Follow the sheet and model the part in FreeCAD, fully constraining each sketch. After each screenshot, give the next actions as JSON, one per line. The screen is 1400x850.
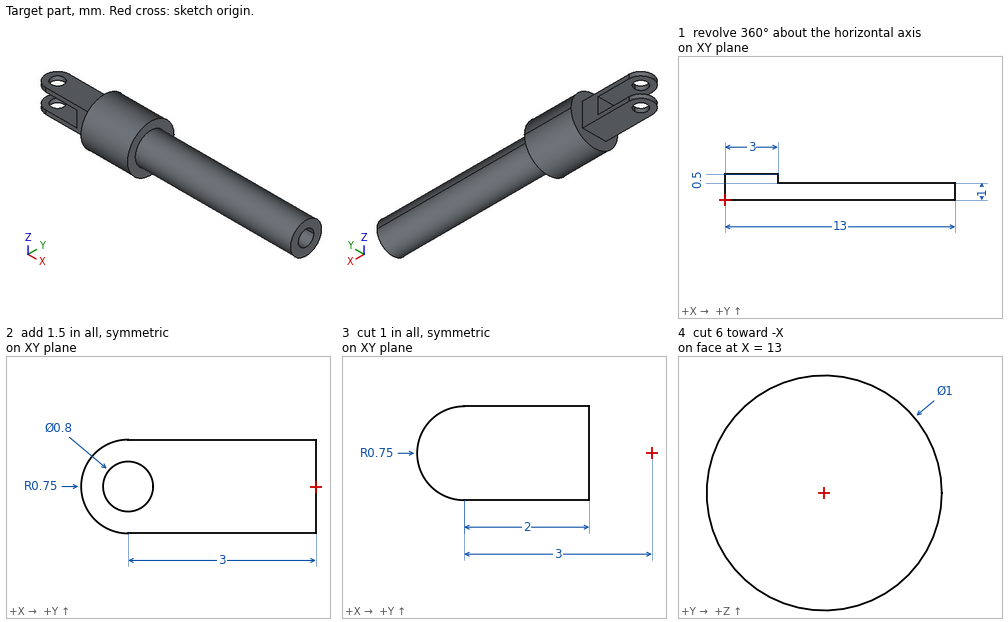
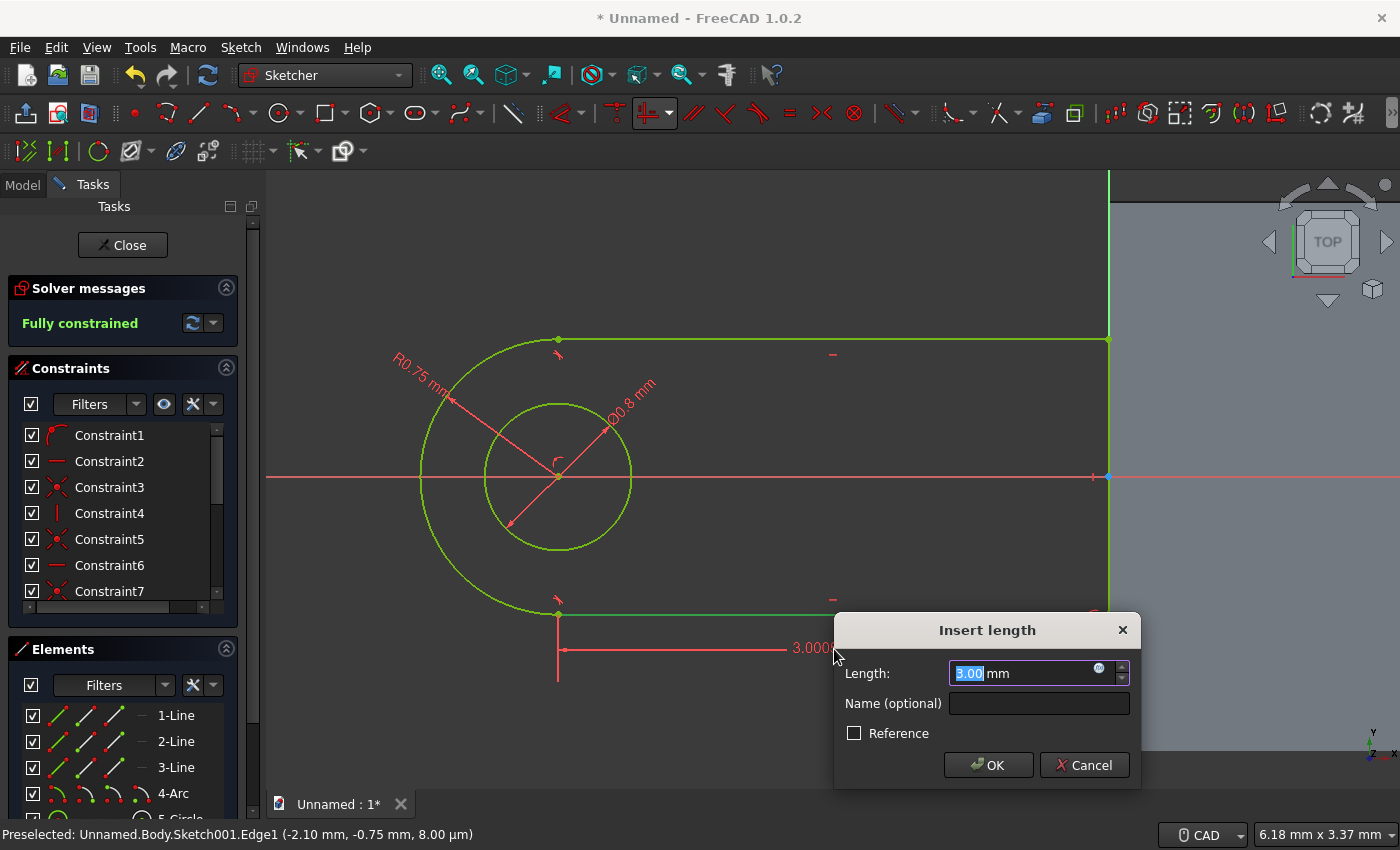
{"action": "type", "text": "3"}
{"action": "key", "text": "Return"}
{"action": "key", "text": "Escape"}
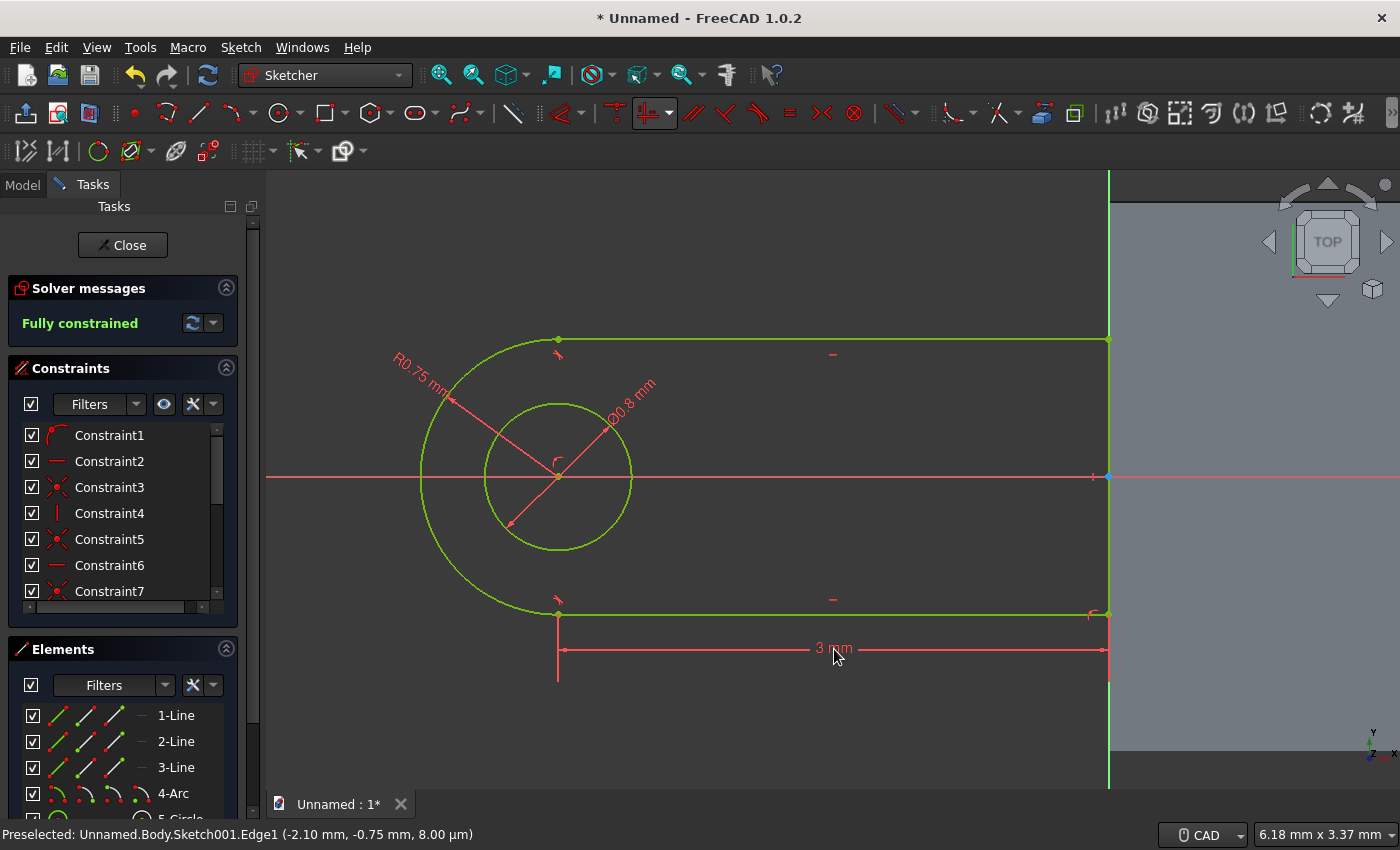
{"action": "left_click", "coordinate": [123, 245]}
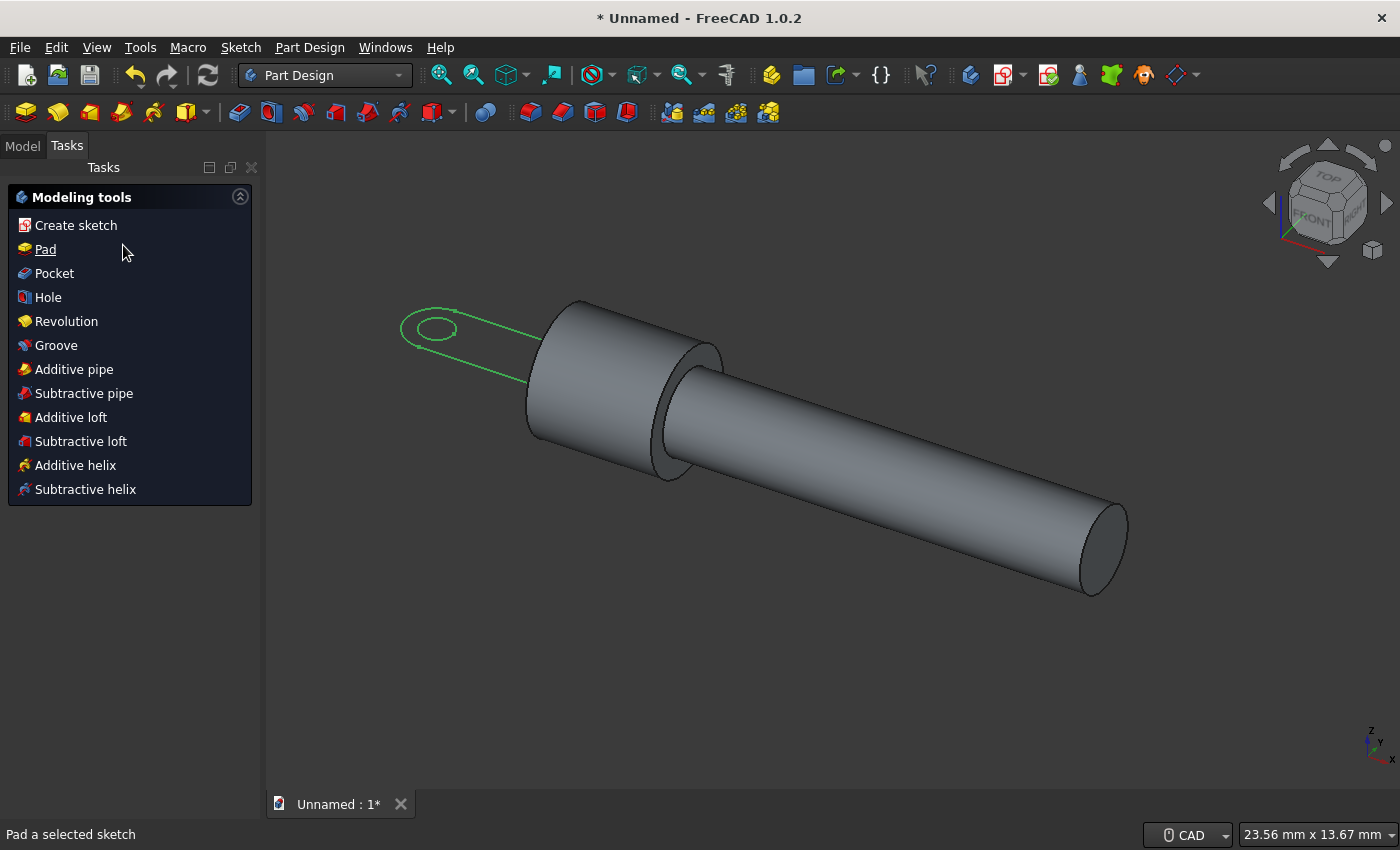
{"action": "left_click", "coordinate": [26, 112]}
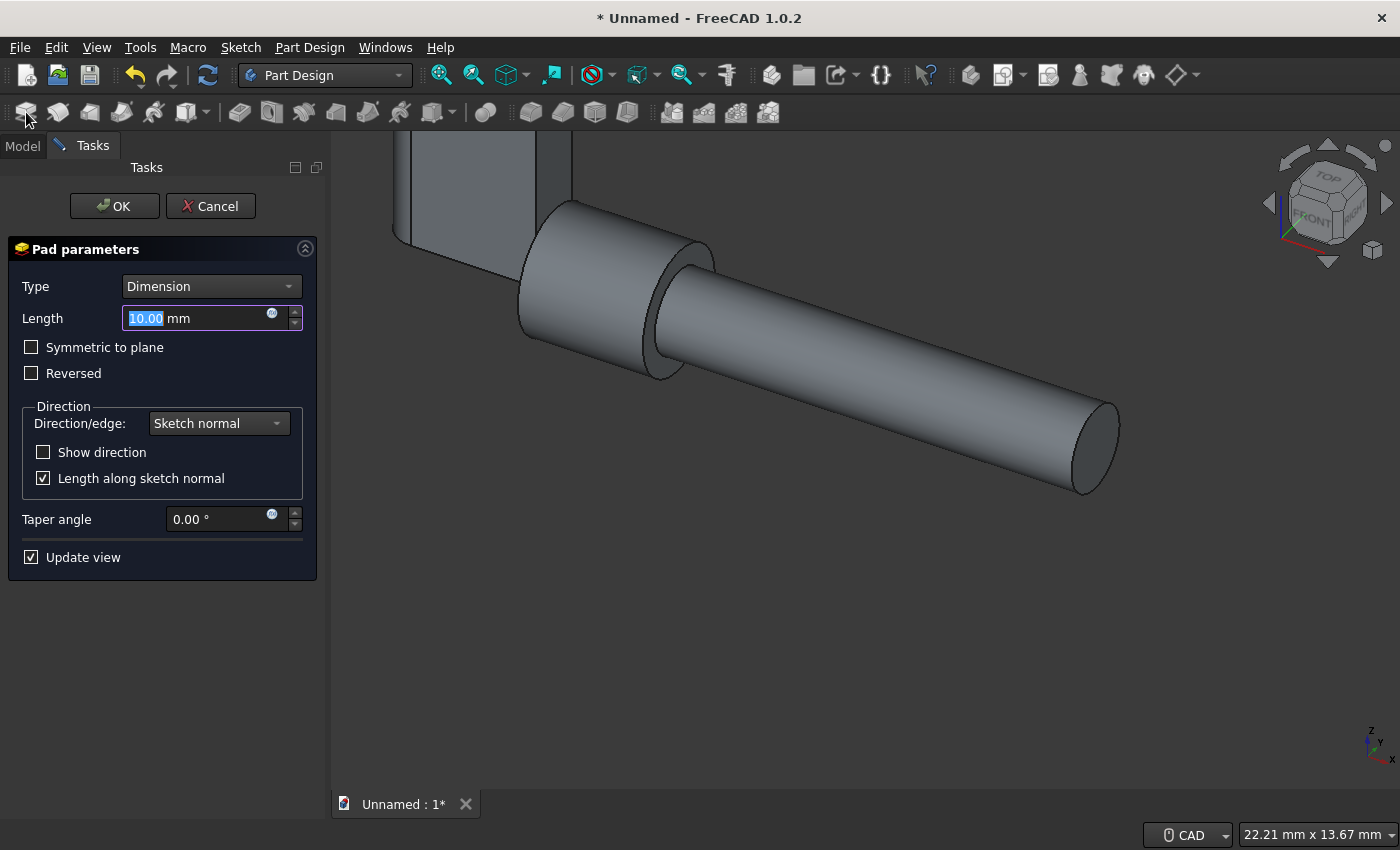
{"action": "type", "text": "1.5"}
{"action": "key", "text": "Tab"}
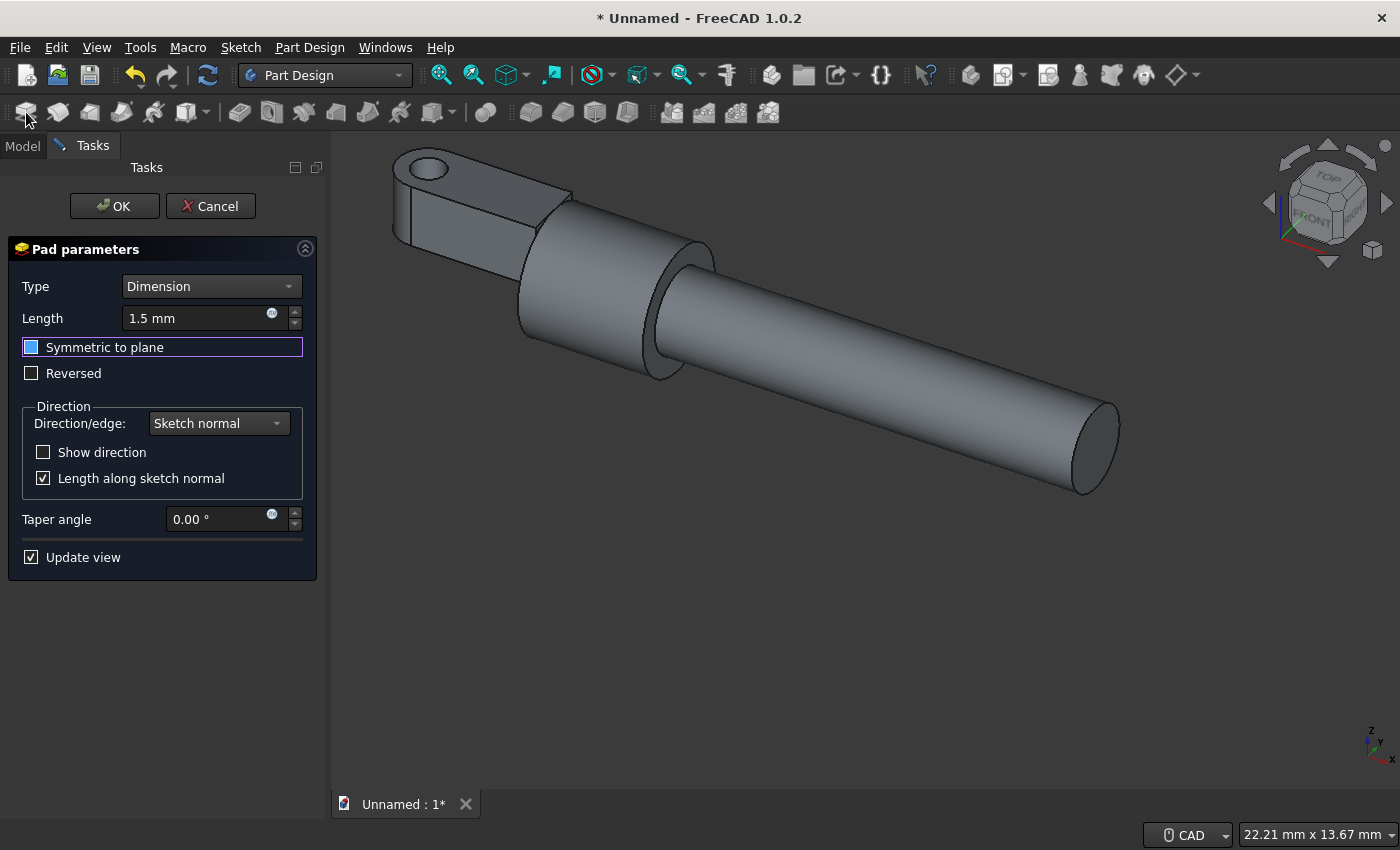
{"action": "left_click", "coordinate": [30, 347]}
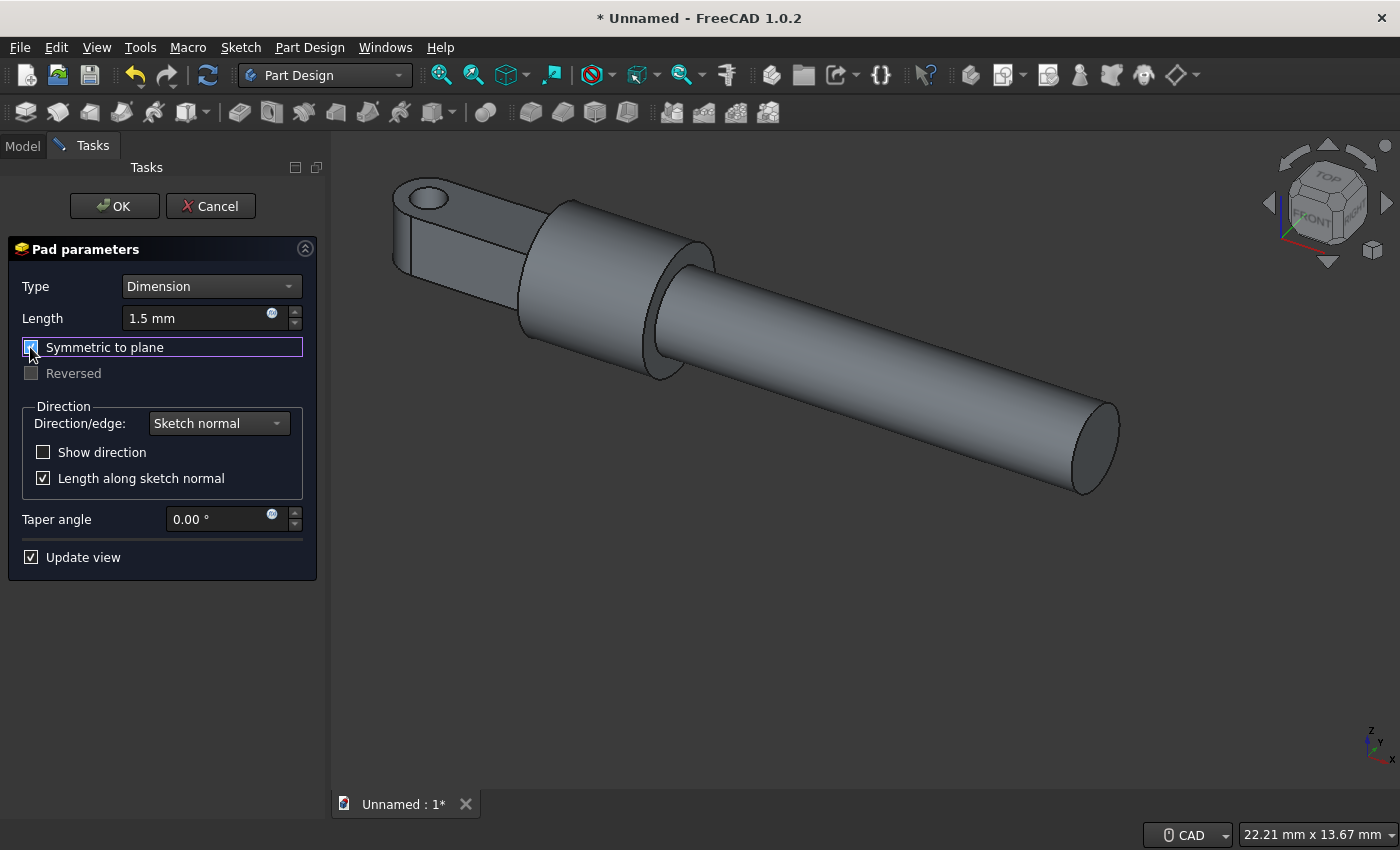
{"action": "left_click", "coordinate": [115, 206]}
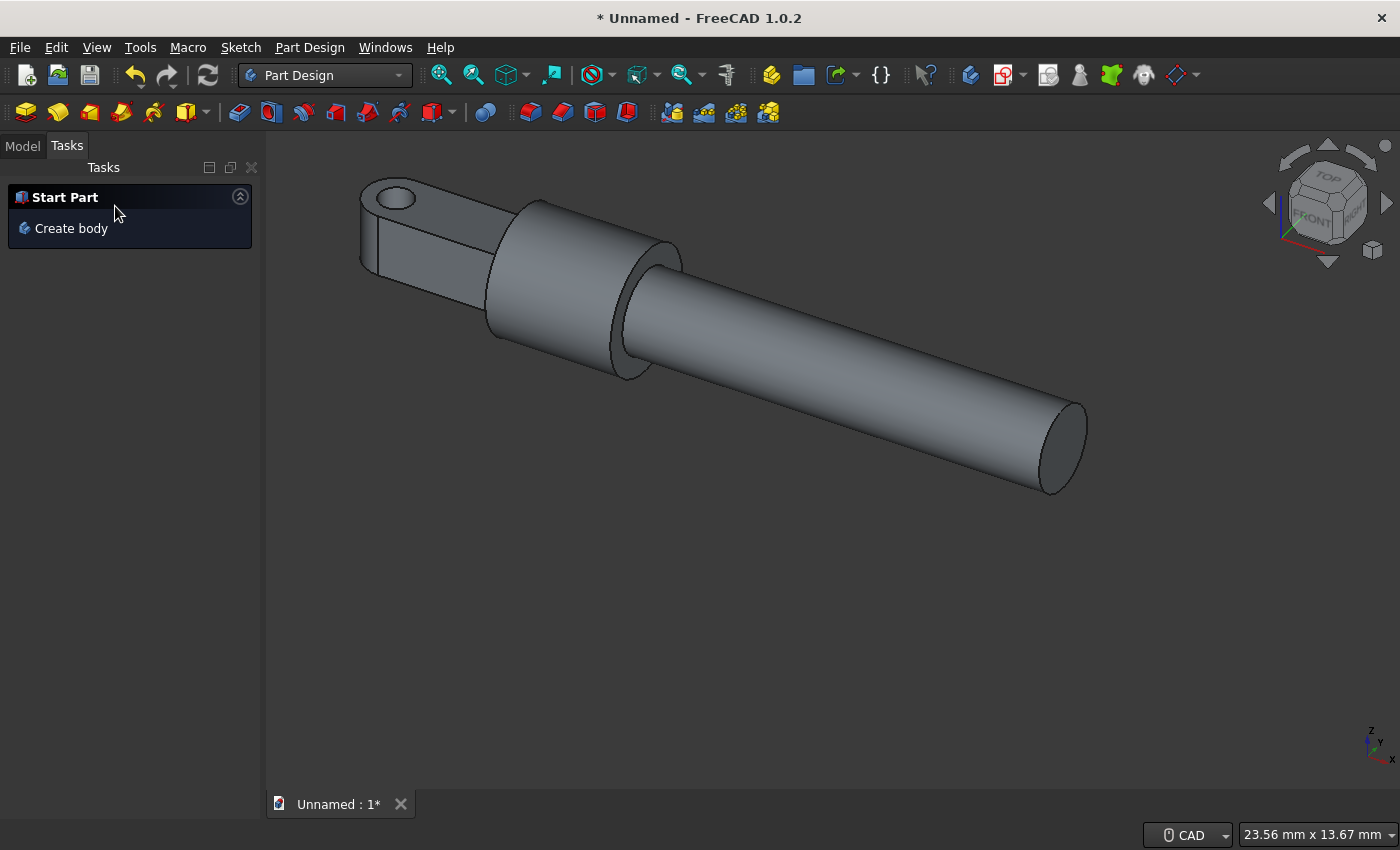
{"action": "left_click", "coordinate": [442, 76]}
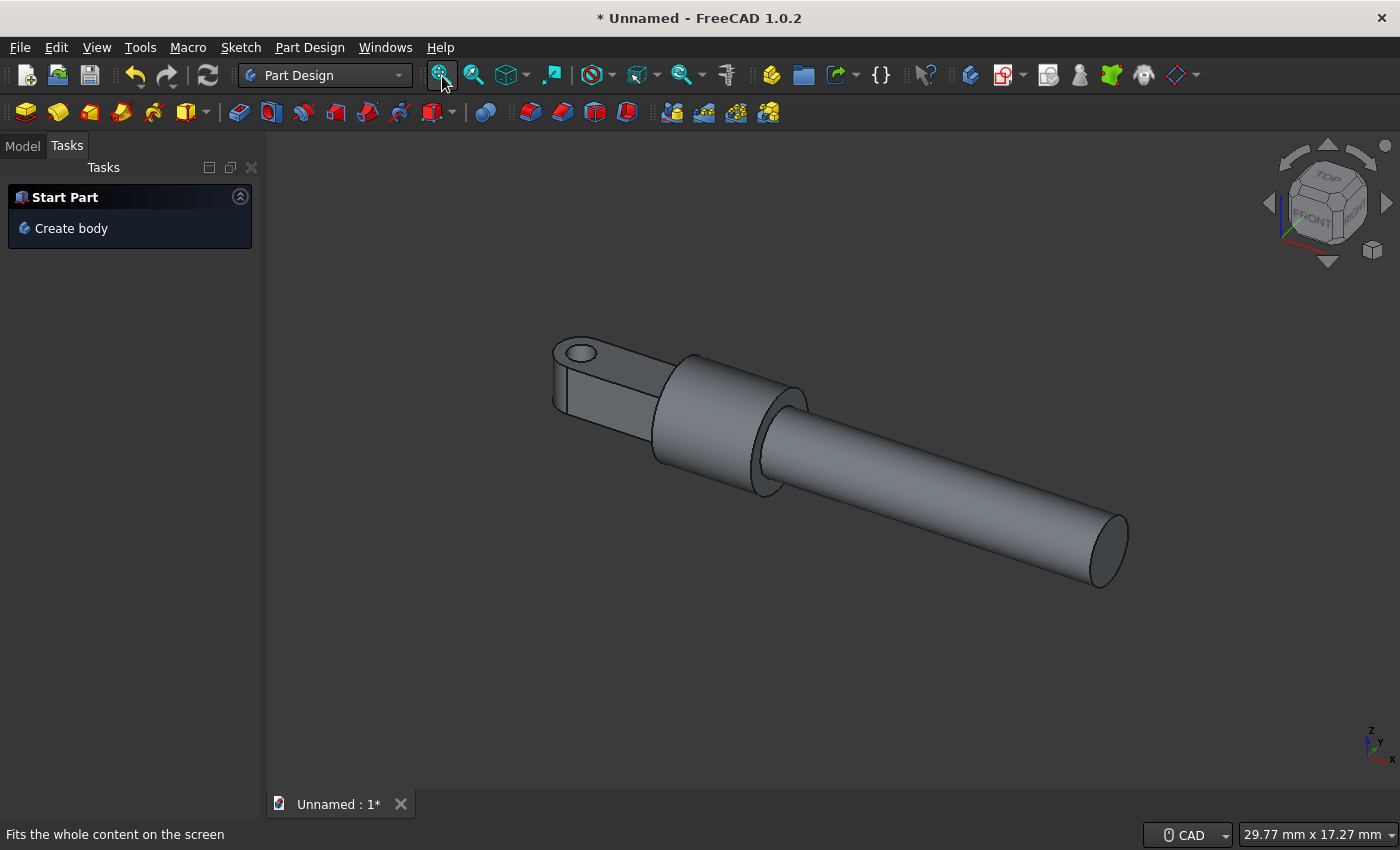
{"action": "left_click", "coordinate": [1004, 76]}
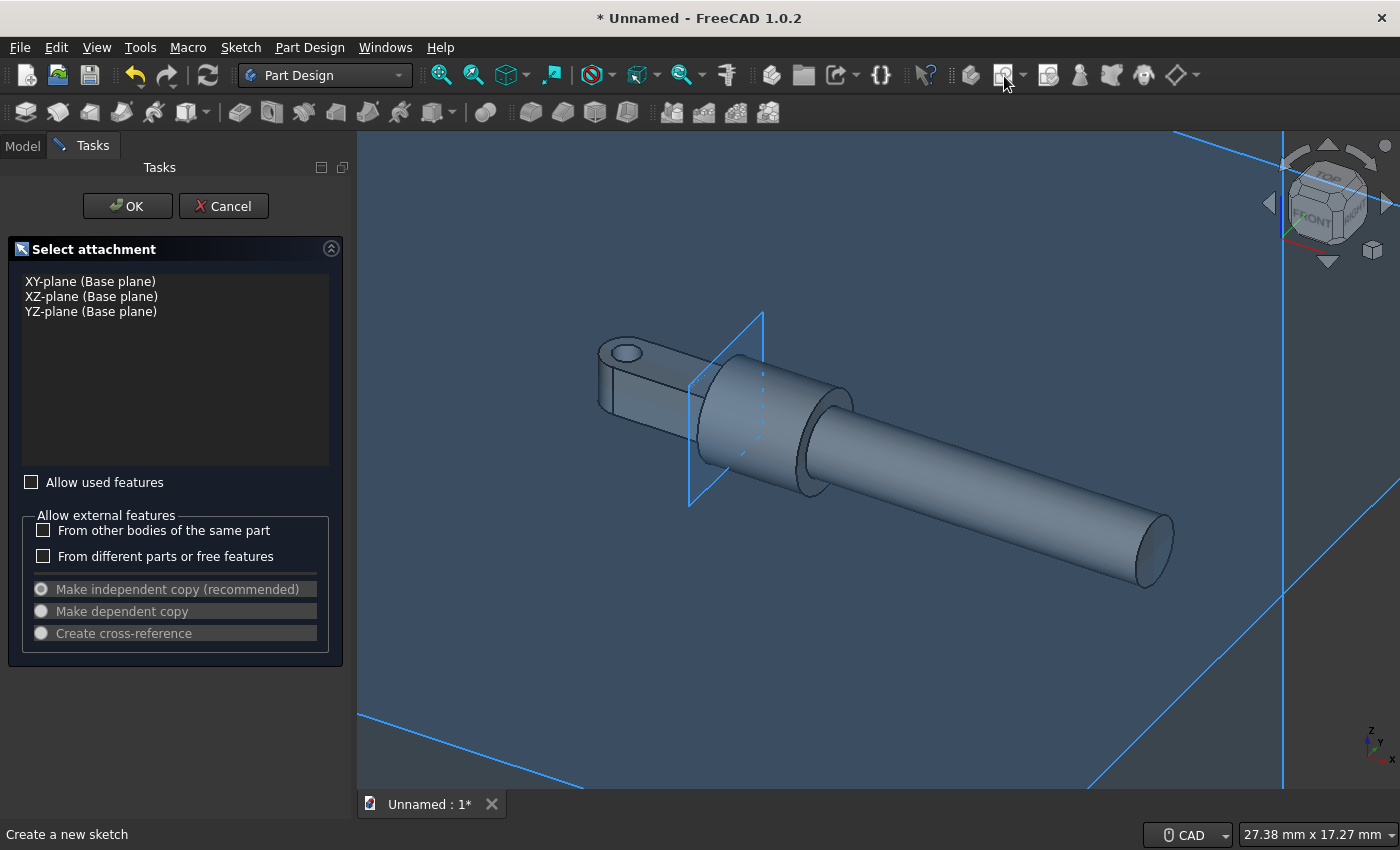
{"action": "left_click", "coordinate": [82, 282]}